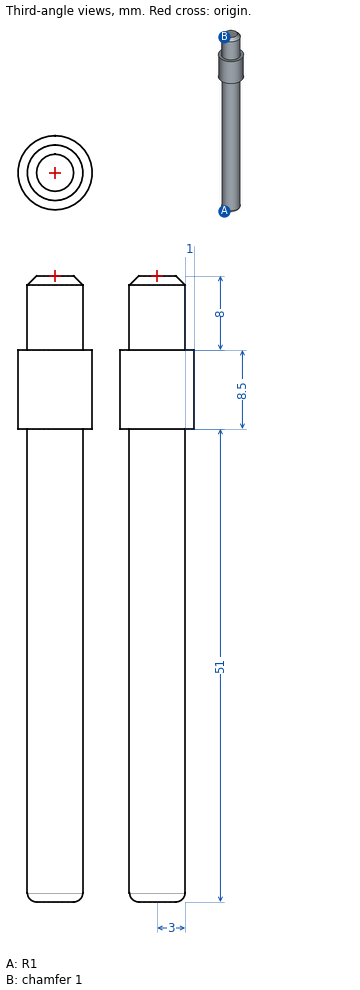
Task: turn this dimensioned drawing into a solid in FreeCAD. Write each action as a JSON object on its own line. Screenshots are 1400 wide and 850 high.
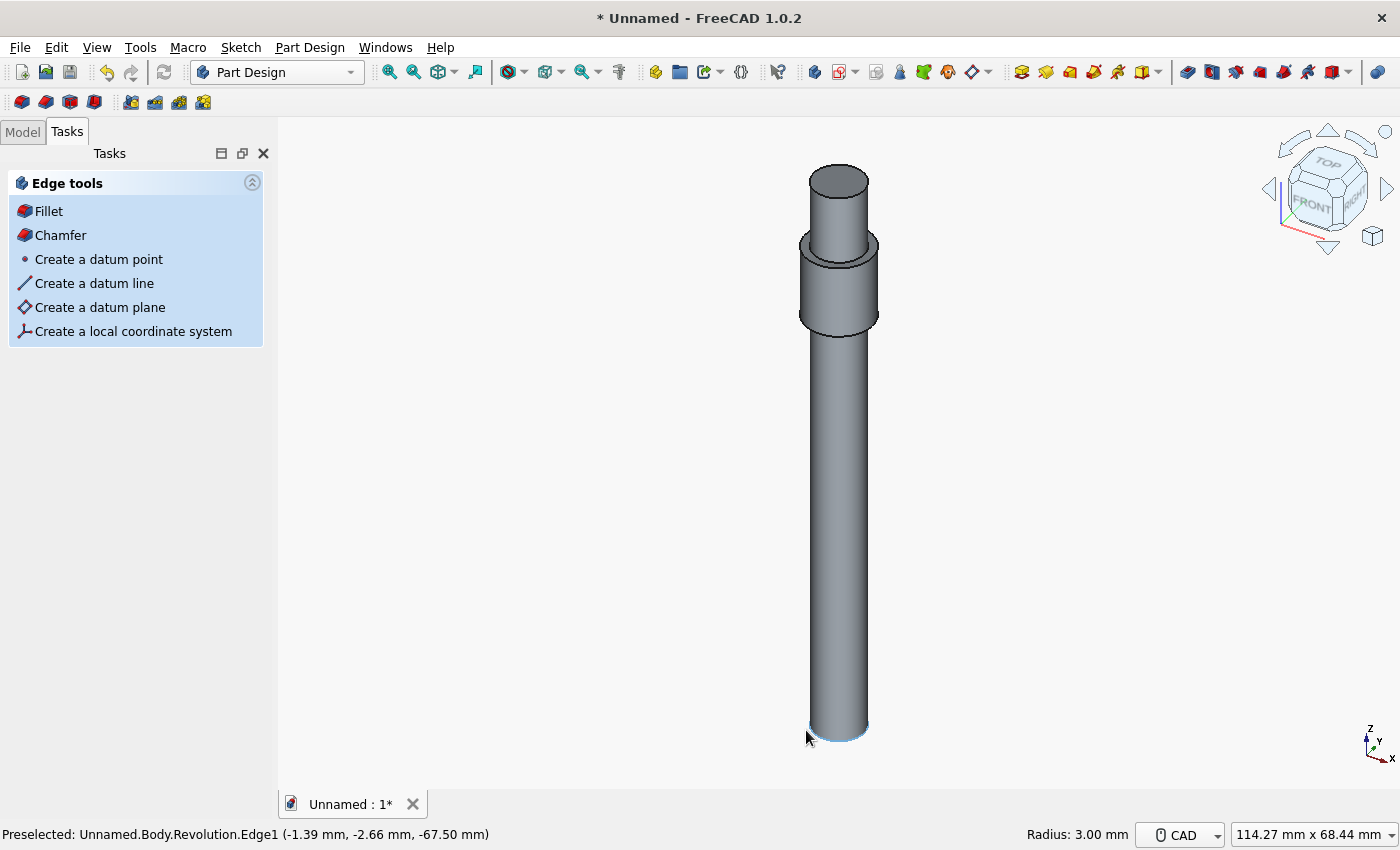
{"action": "left_click", "coordinate": [22, 102]}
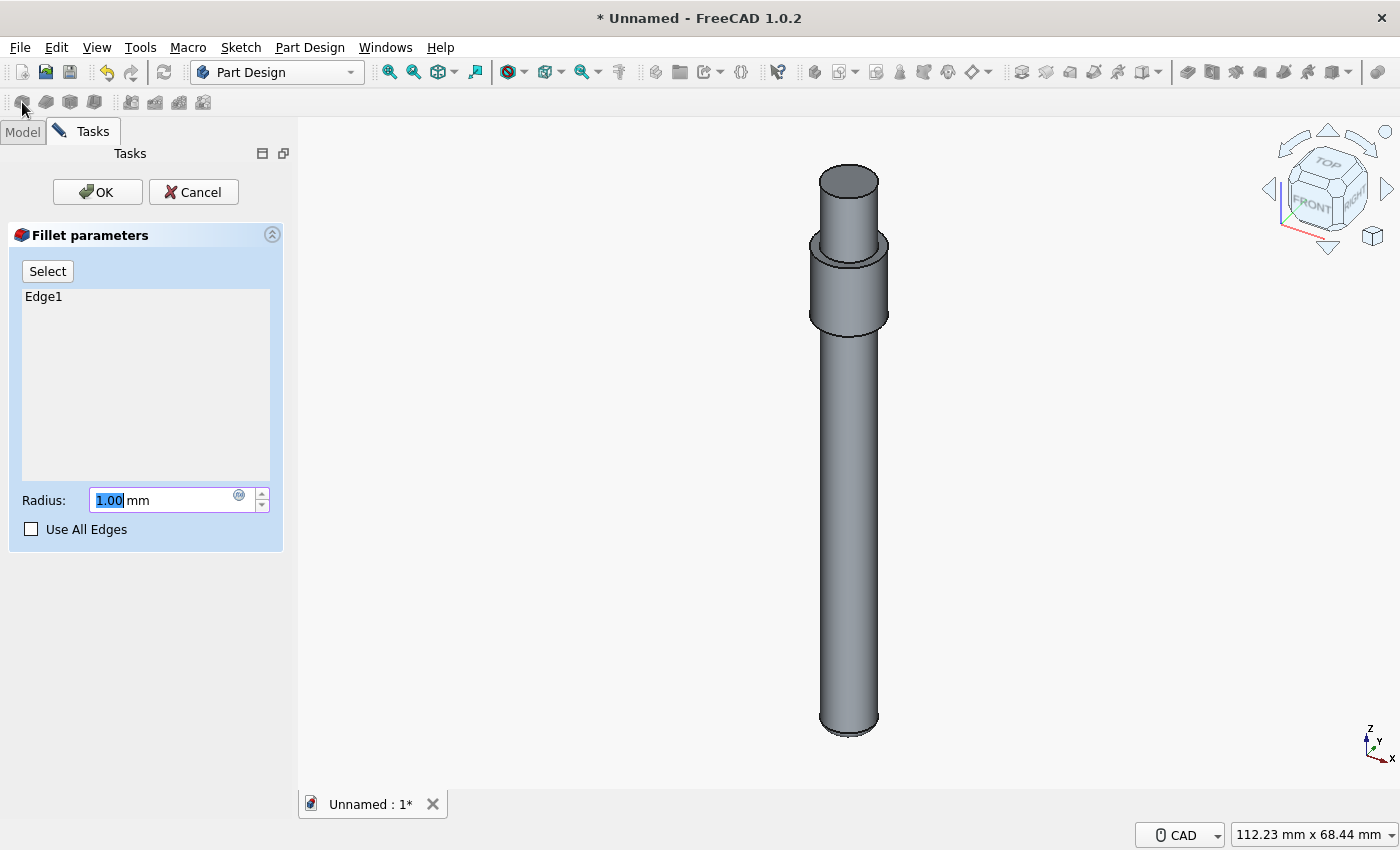
{"action": "type", "text": "1"}
{"action": "key", "text": "Tab"}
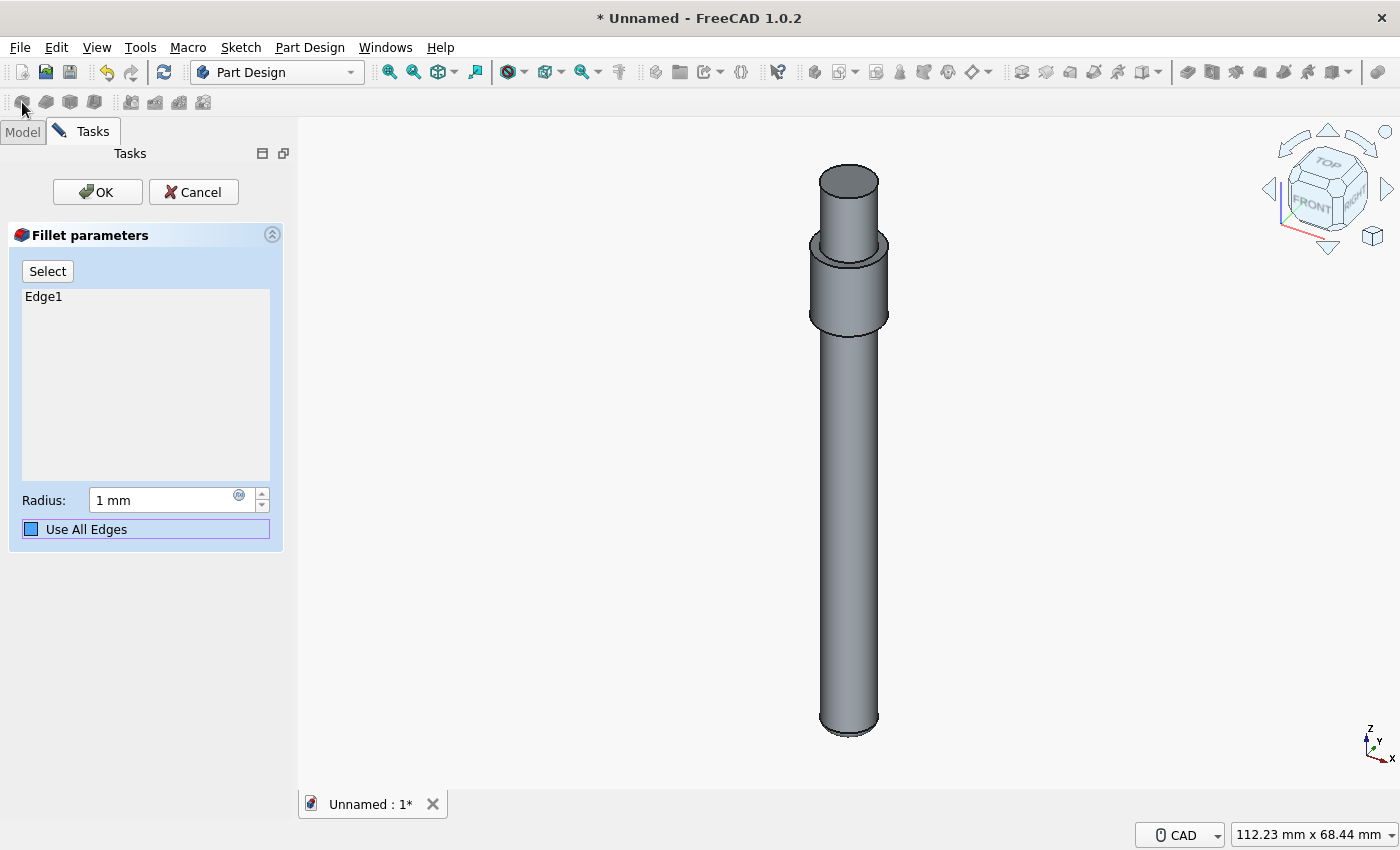
{"action": "left_click", "coordinate": [98, 192]}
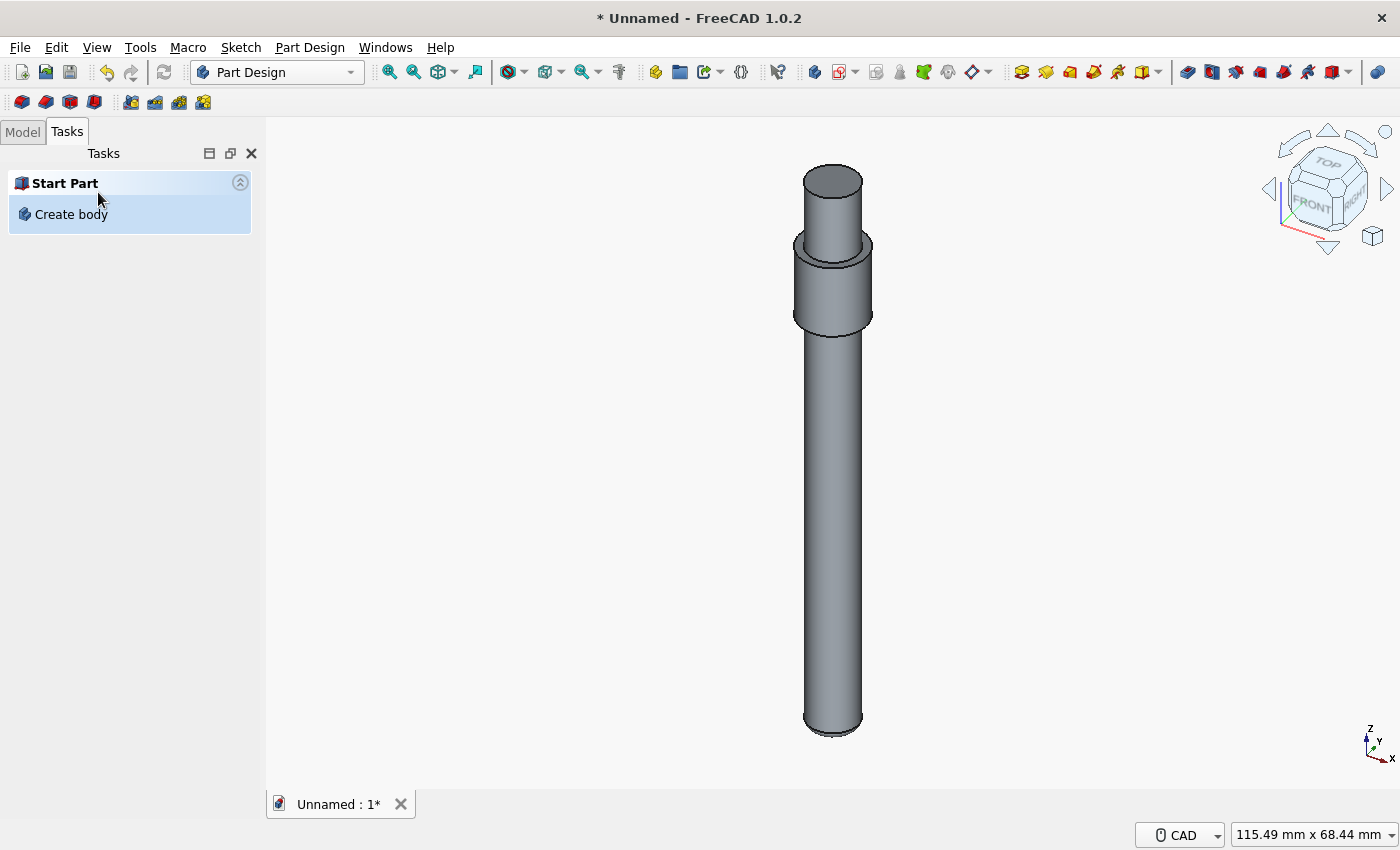
{"action": "left_click", "coordinate": [818, 195]}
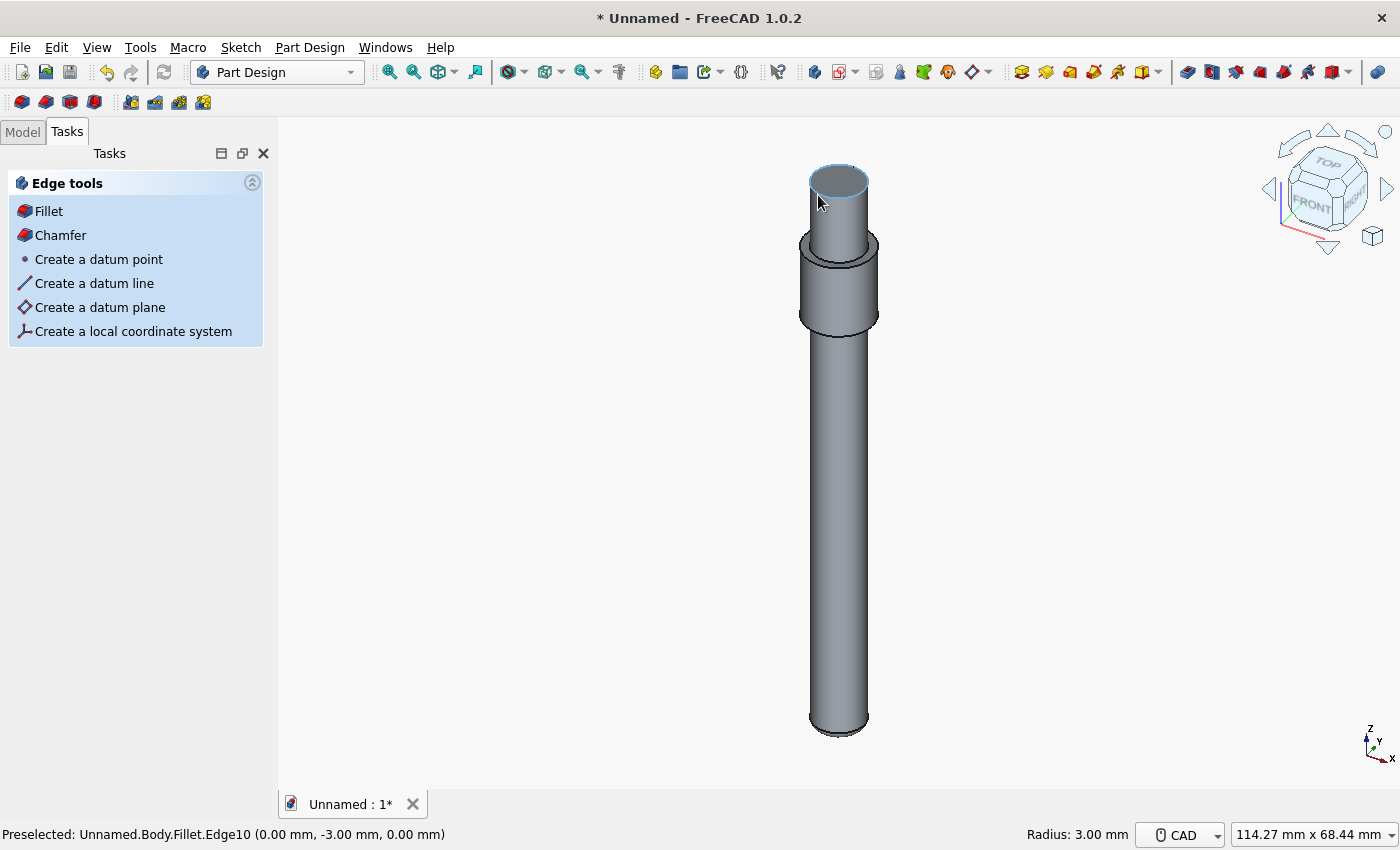
{"action": "left_click", "coordinate": [46, 102]}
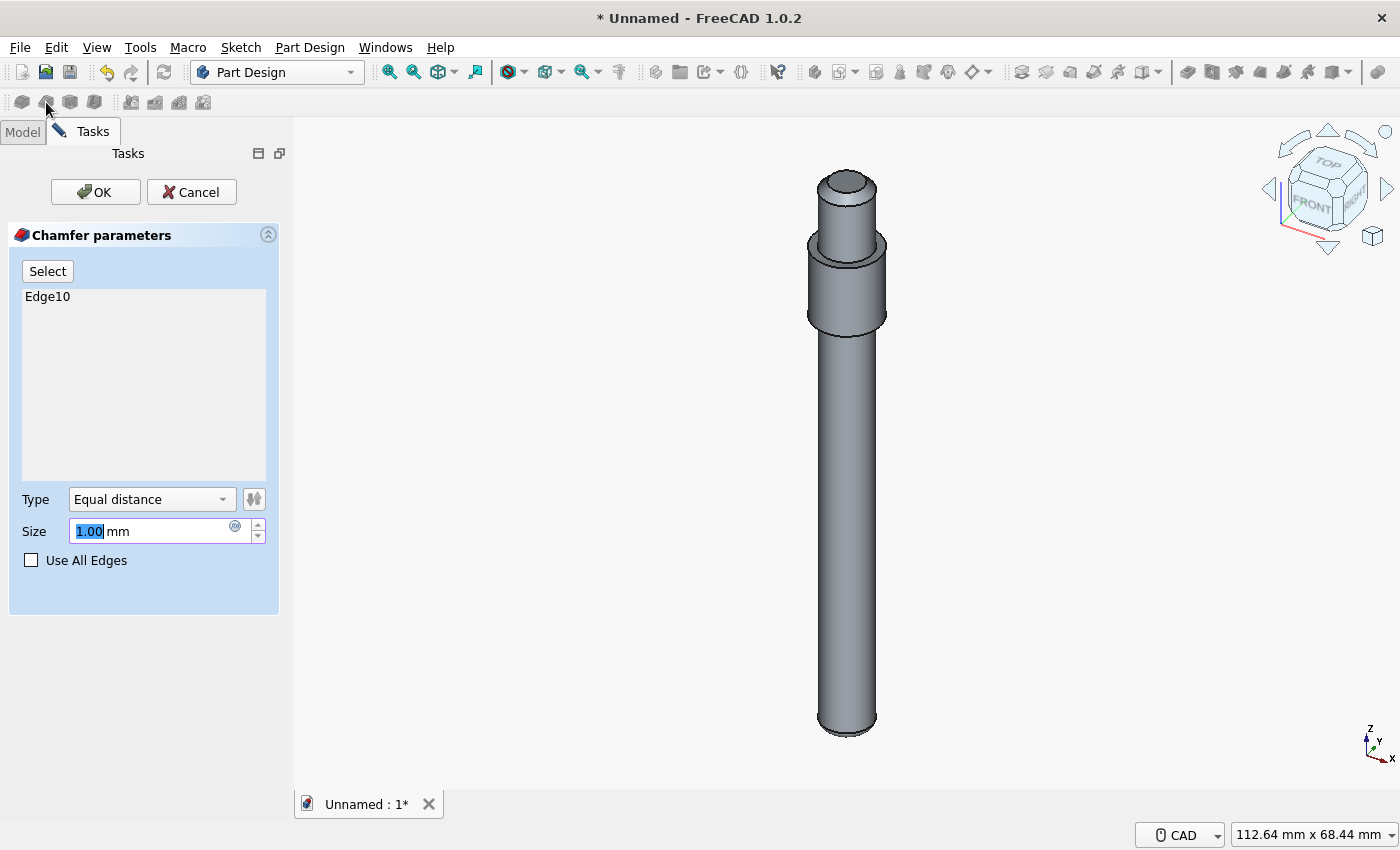
{"action": "type", "text": "1"}
{"action": "key", "text": "Tab"}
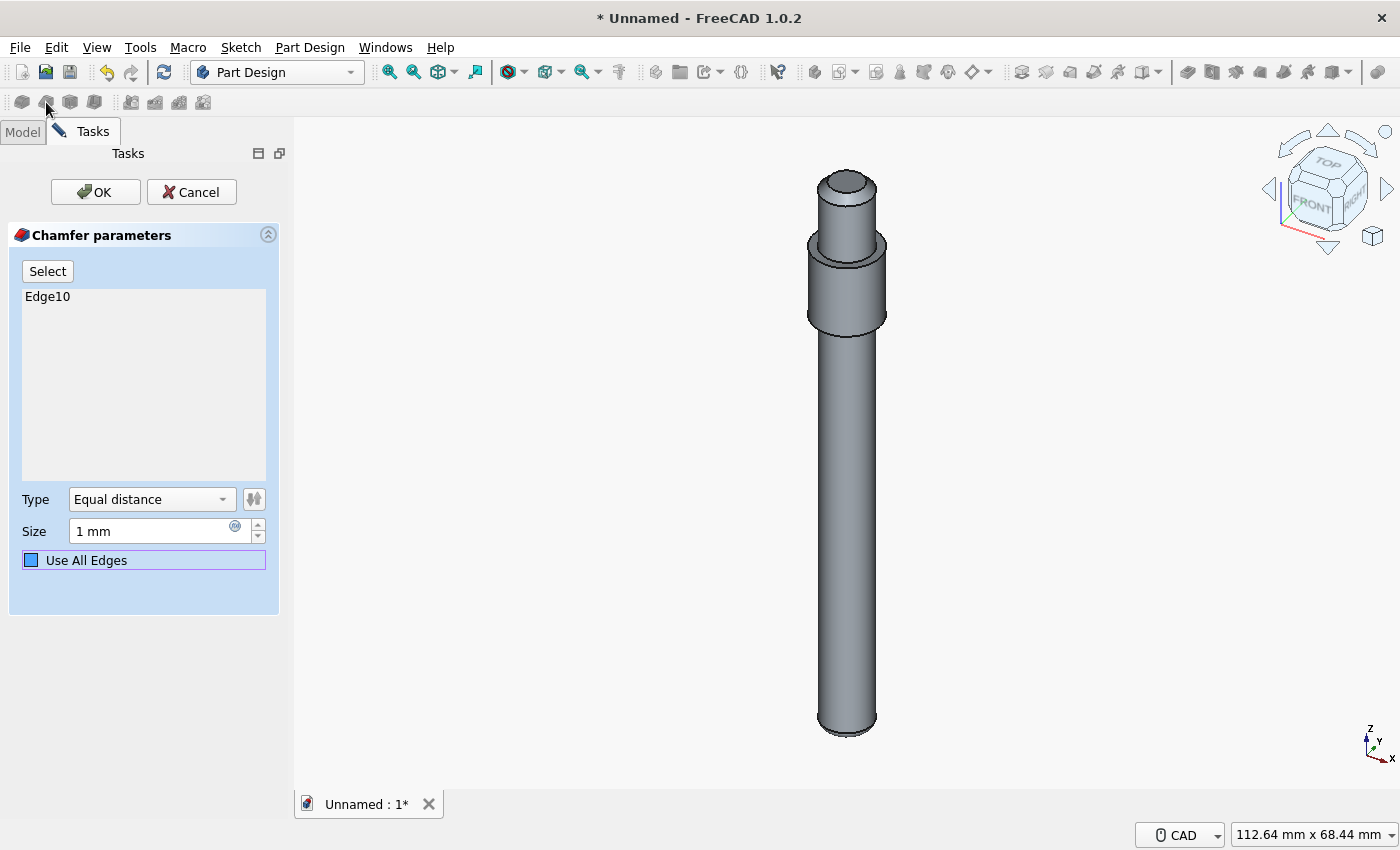
{"action": "left_click", "coordinate": [96, 192]}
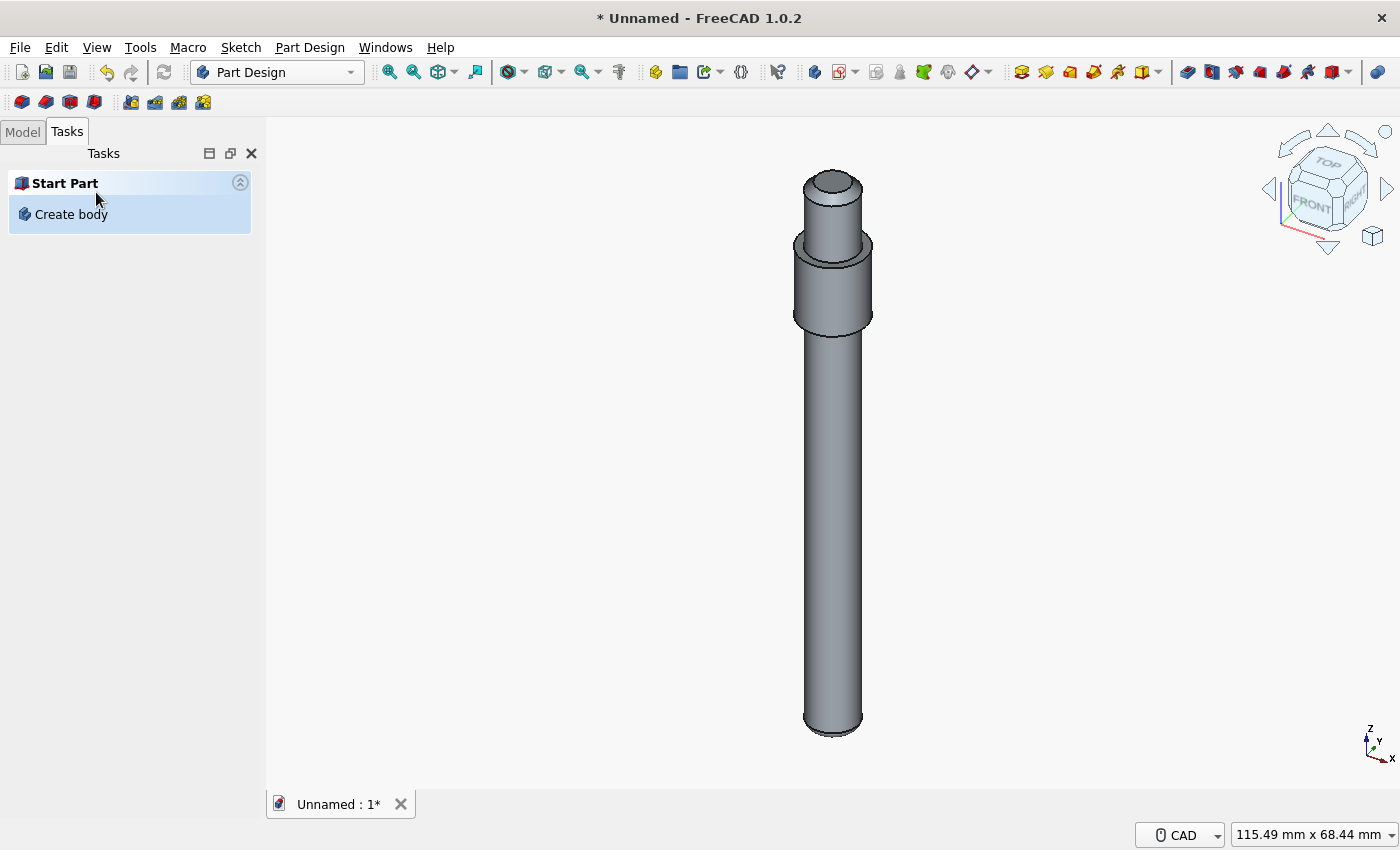
{"action": "key", "text": "0"}